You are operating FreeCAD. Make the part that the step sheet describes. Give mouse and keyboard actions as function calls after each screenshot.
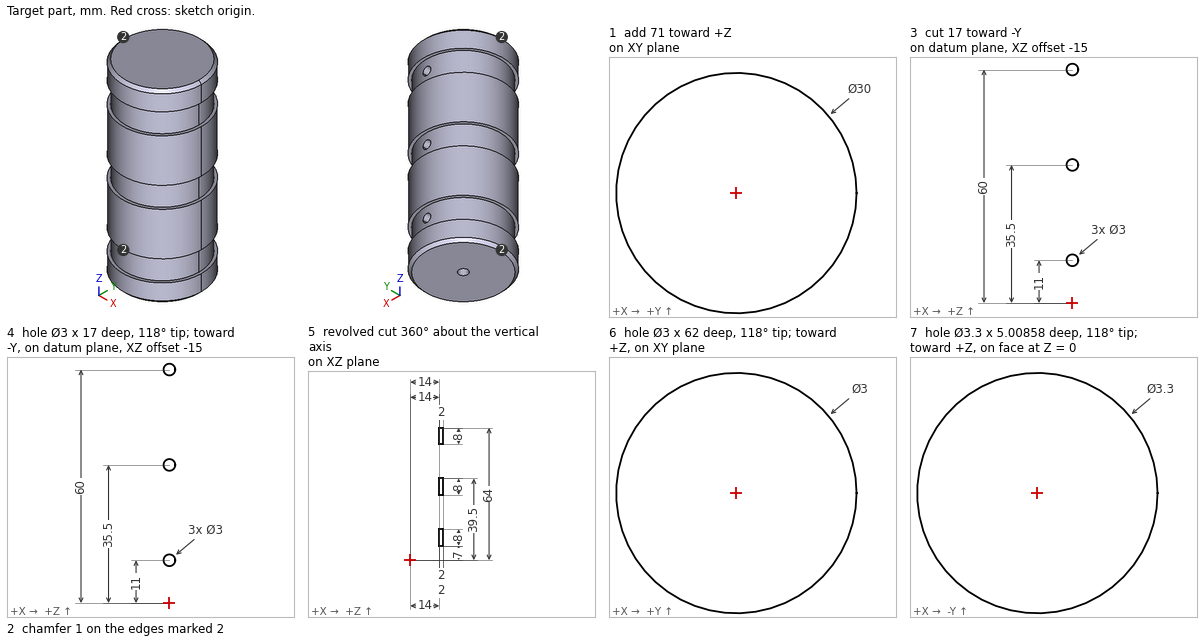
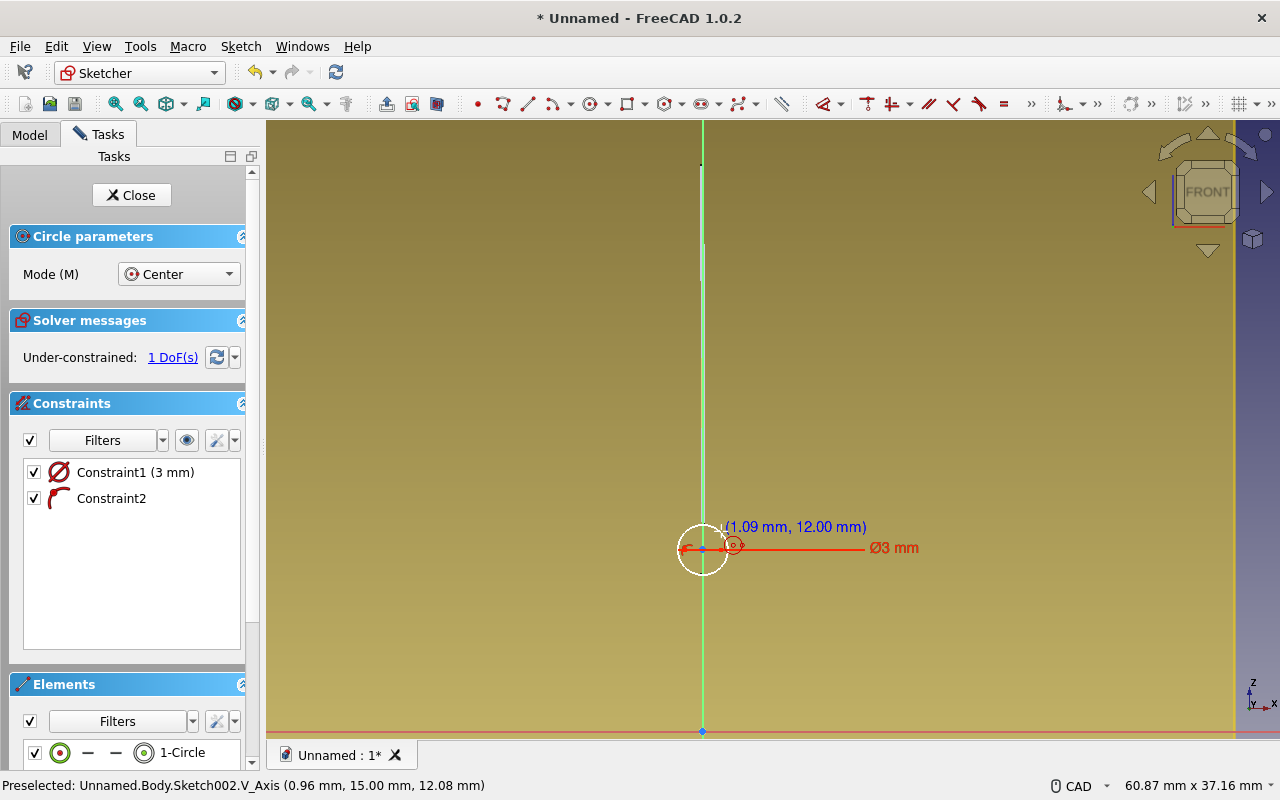
scroll(705, 552, down, 5)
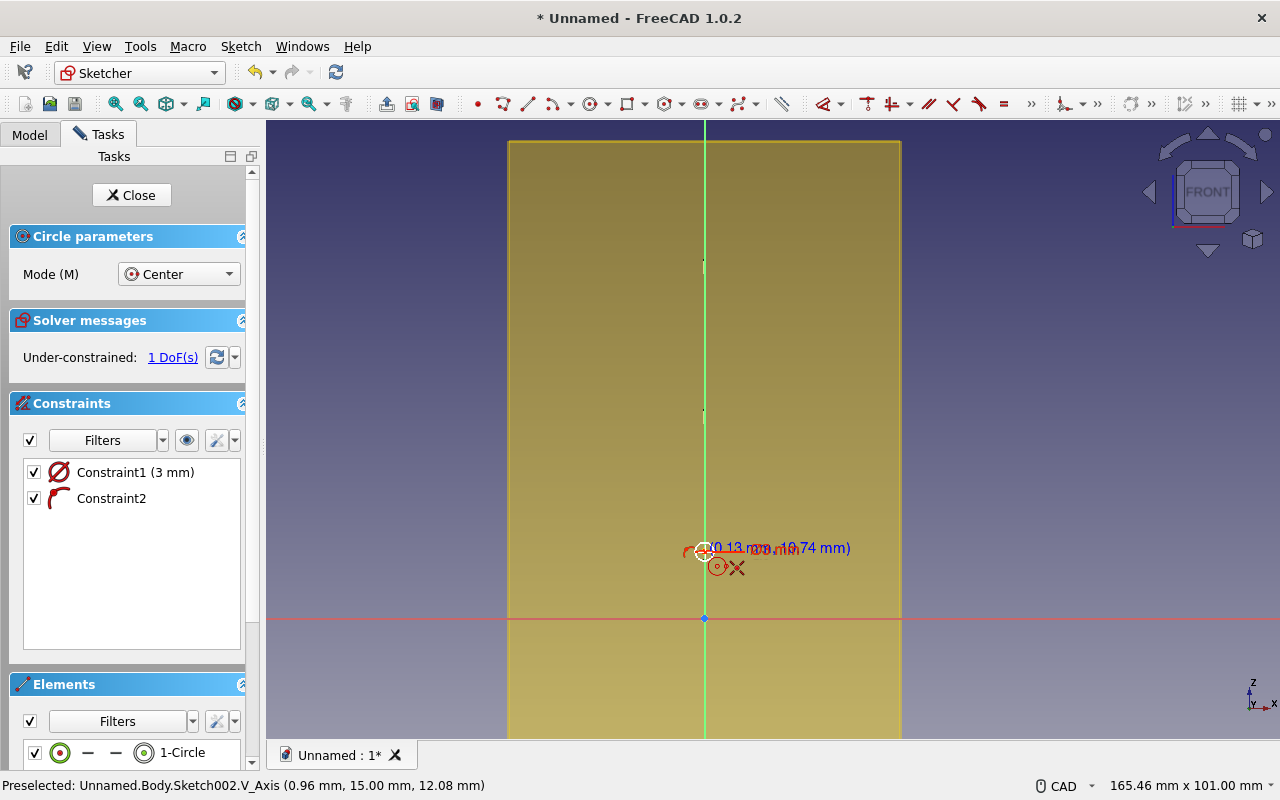
scroll(705, 401, up, 5)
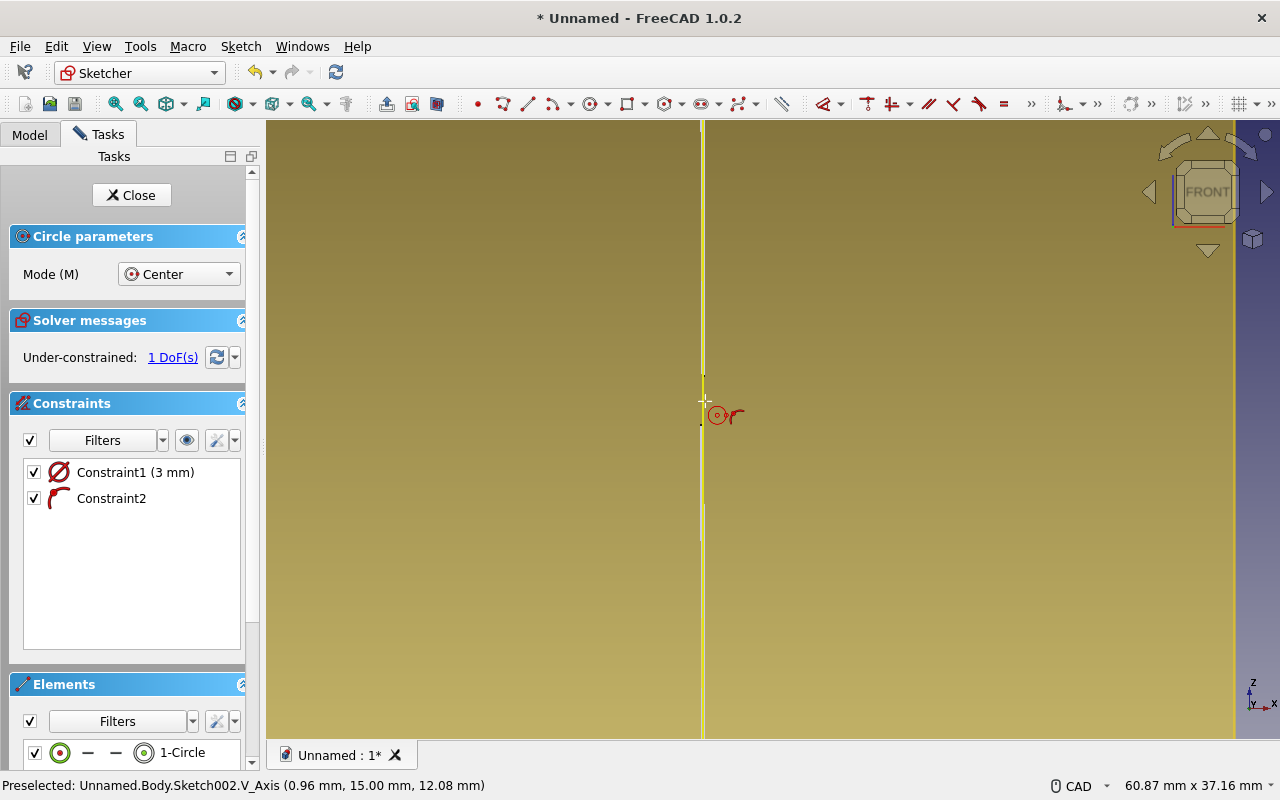
click(703, 400)
move(721, 383)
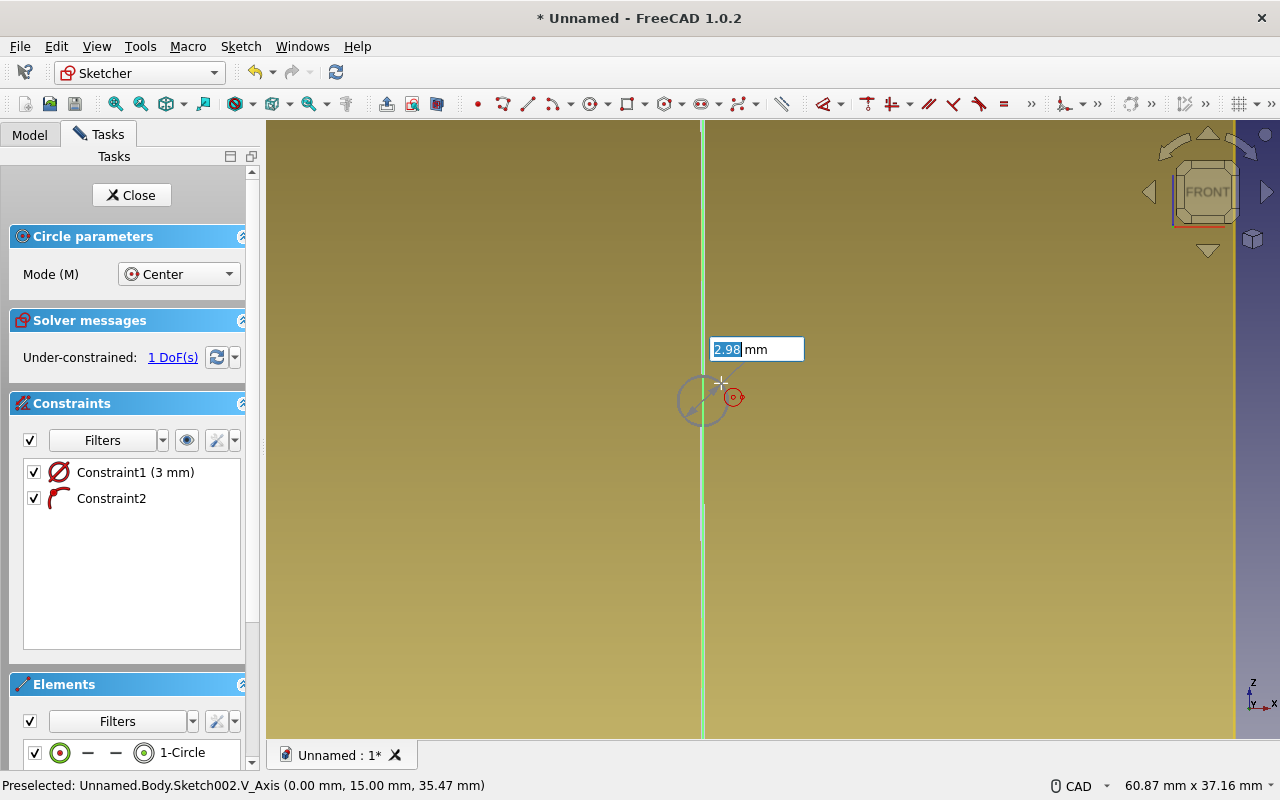
text(3)
key(Return)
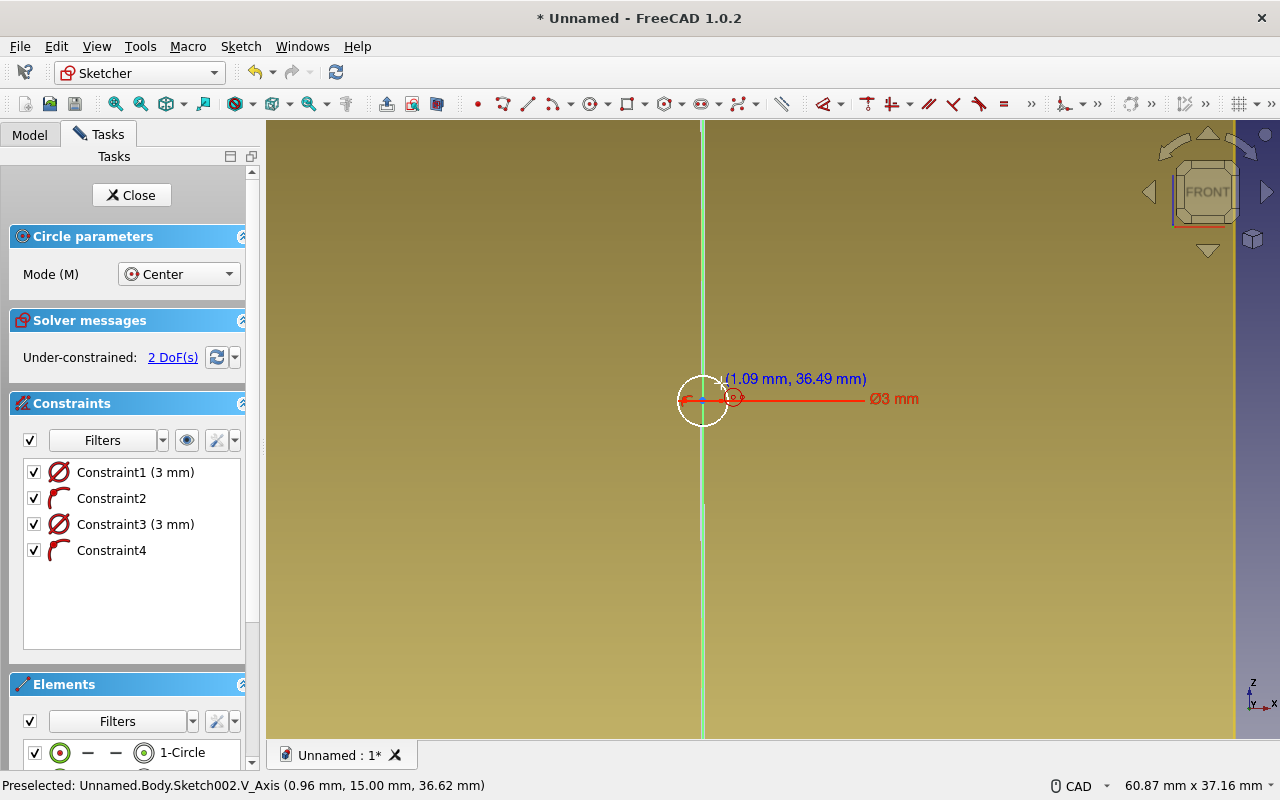
scroll(705, 400, down, 5)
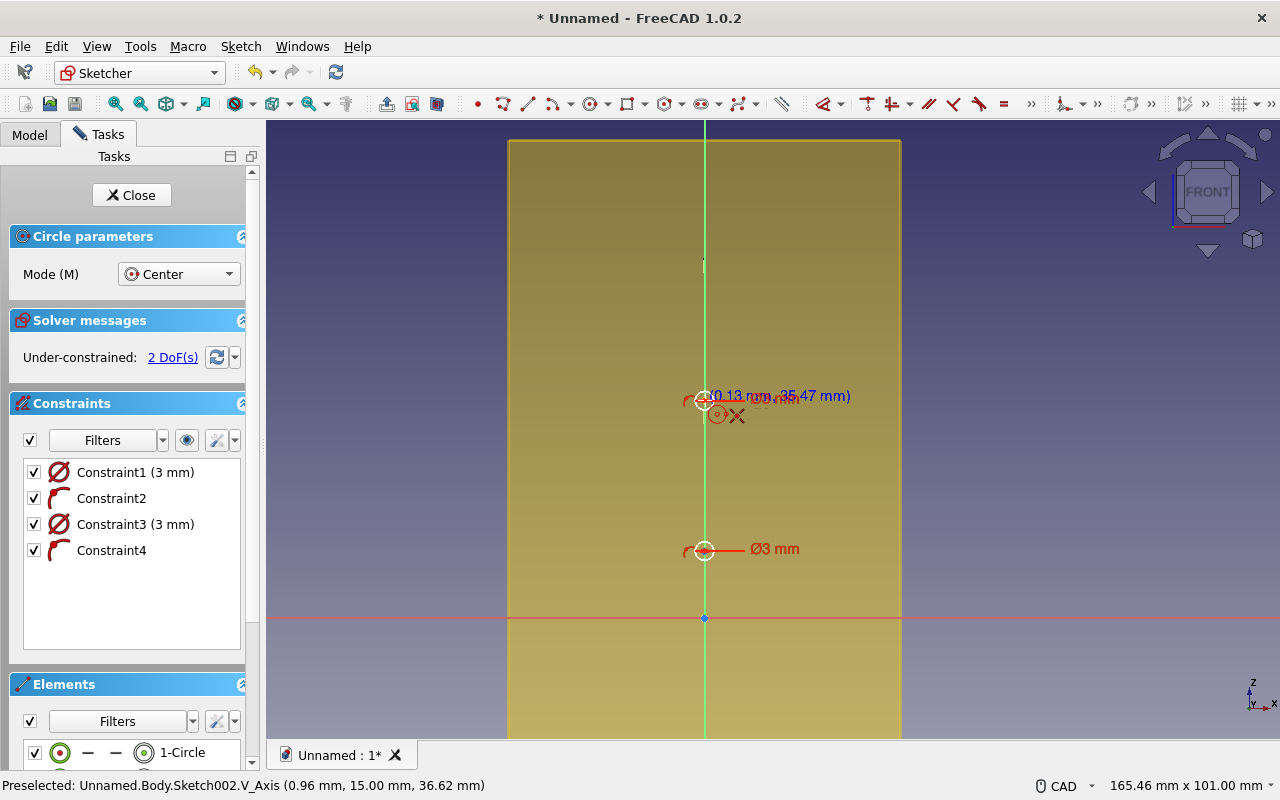
scroll(705, 250, up, 5)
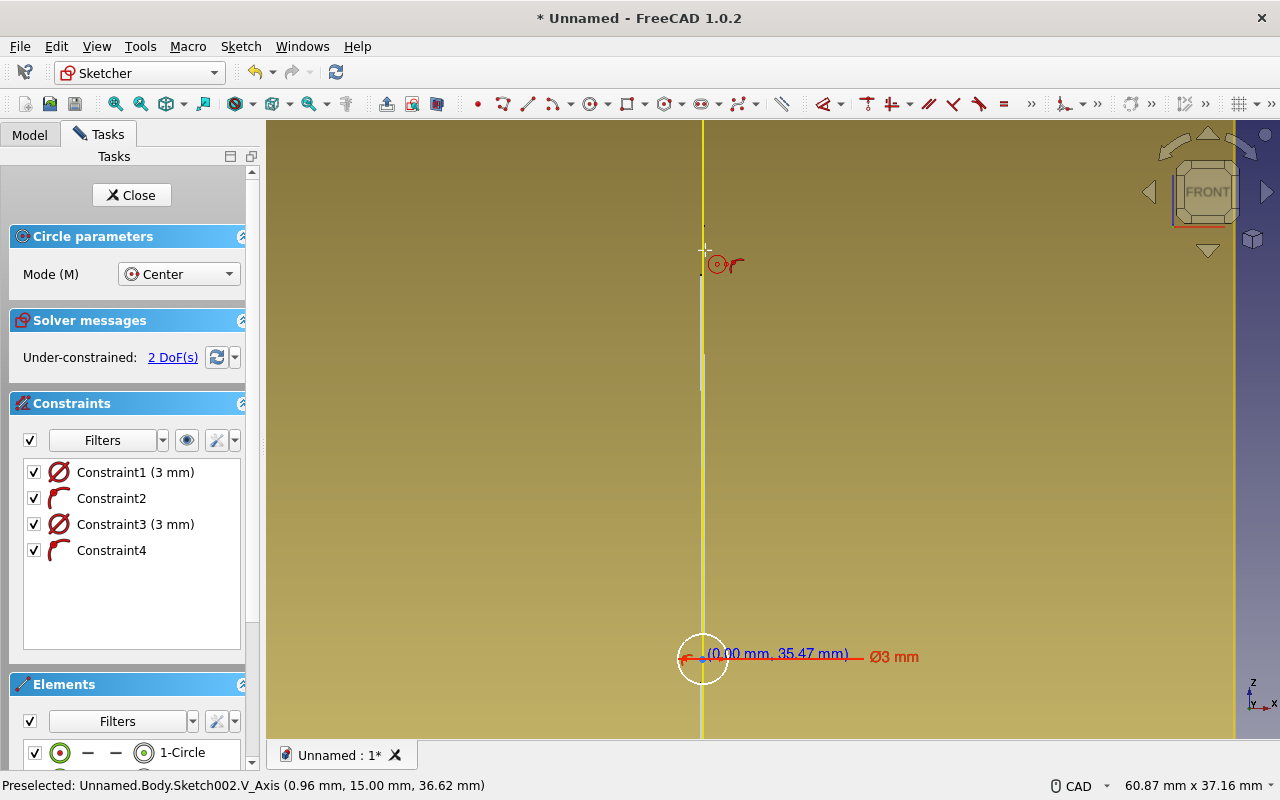
click(703, 250)
move(721, 233)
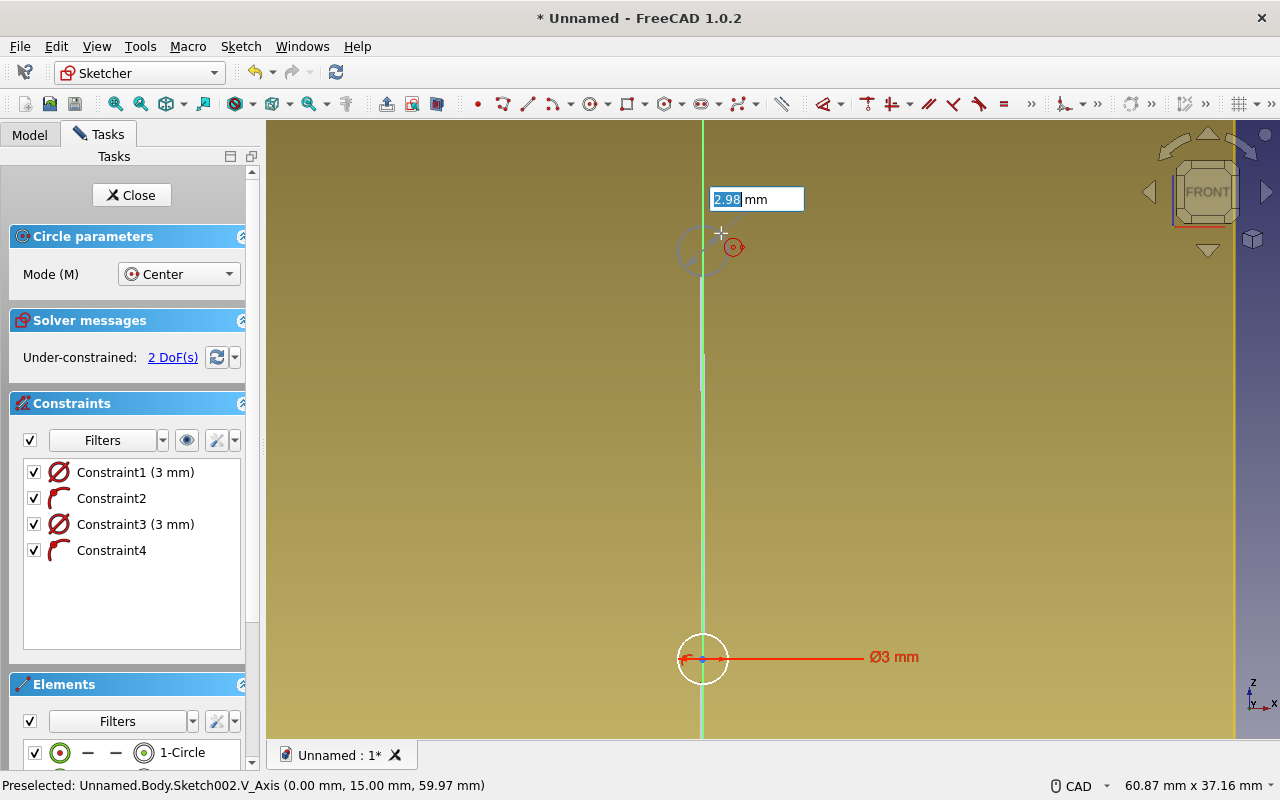
text(3)
key(Return)
key(Escape)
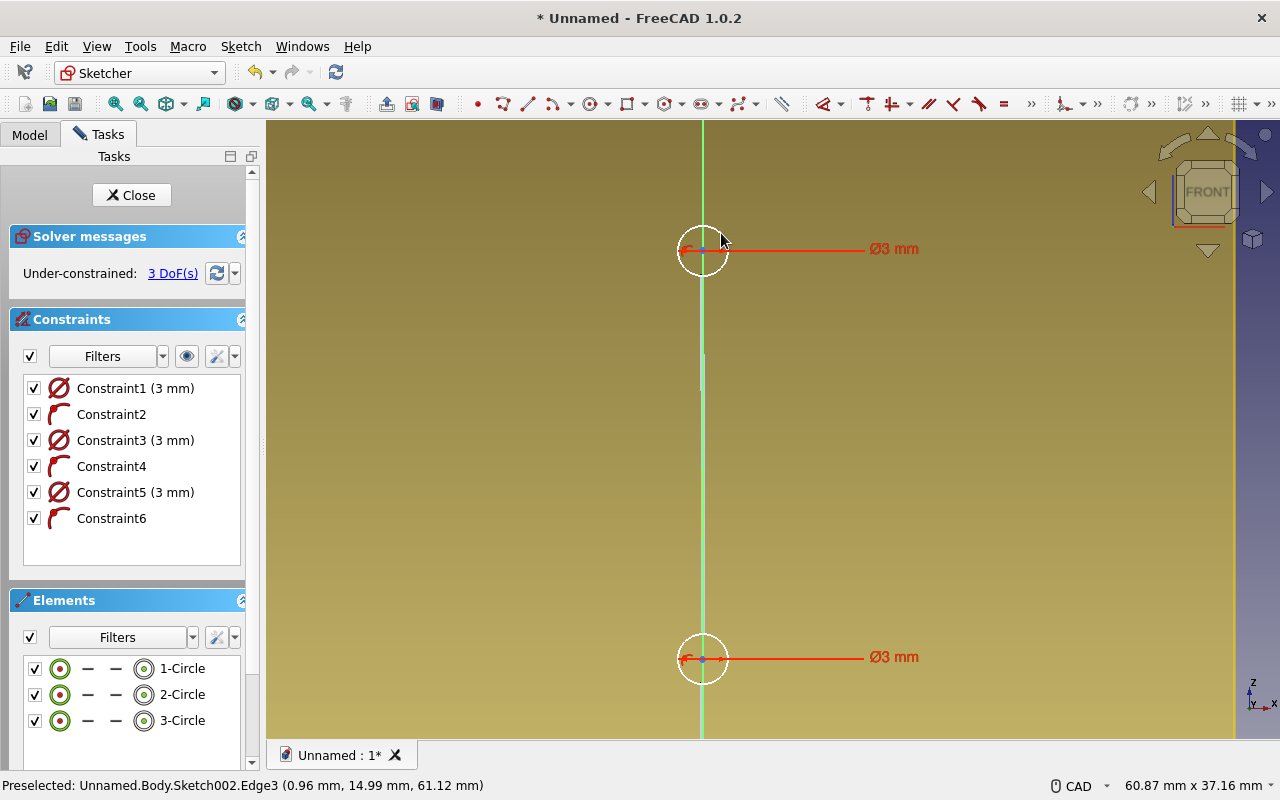
click(822, 104)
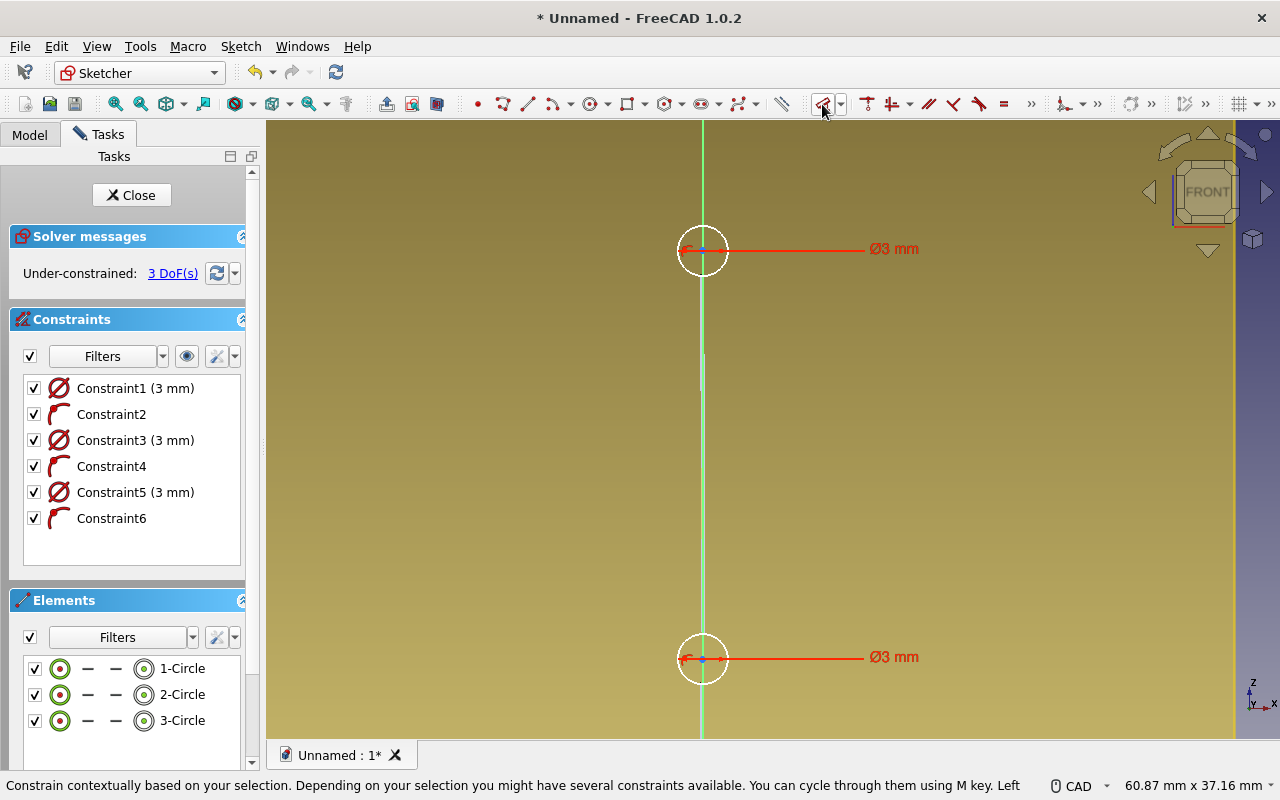
scroll(705, 250, down, 5)